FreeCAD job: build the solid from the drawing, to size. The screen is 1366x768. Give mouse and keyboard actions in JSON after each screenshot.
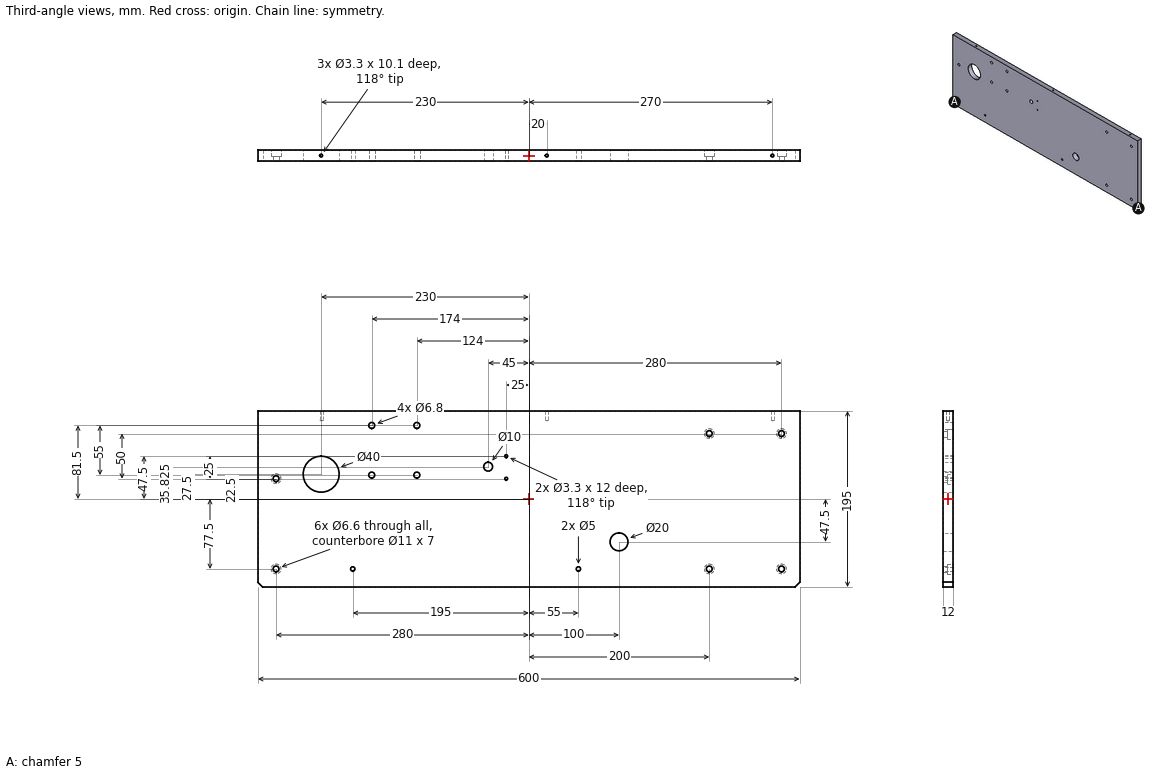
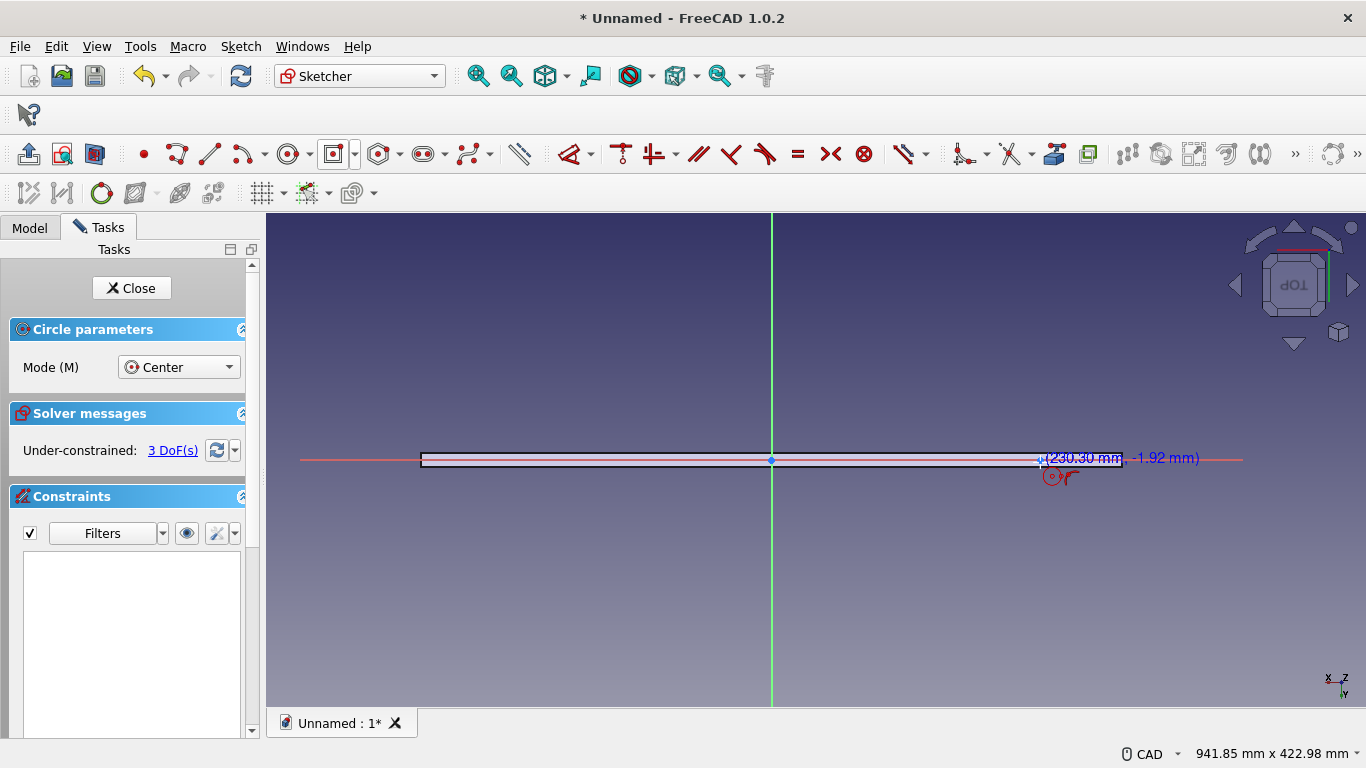
{"action": "scroll", "coordinate": [748, 460], "scroll_direction": "up", "scroll_amount": 13}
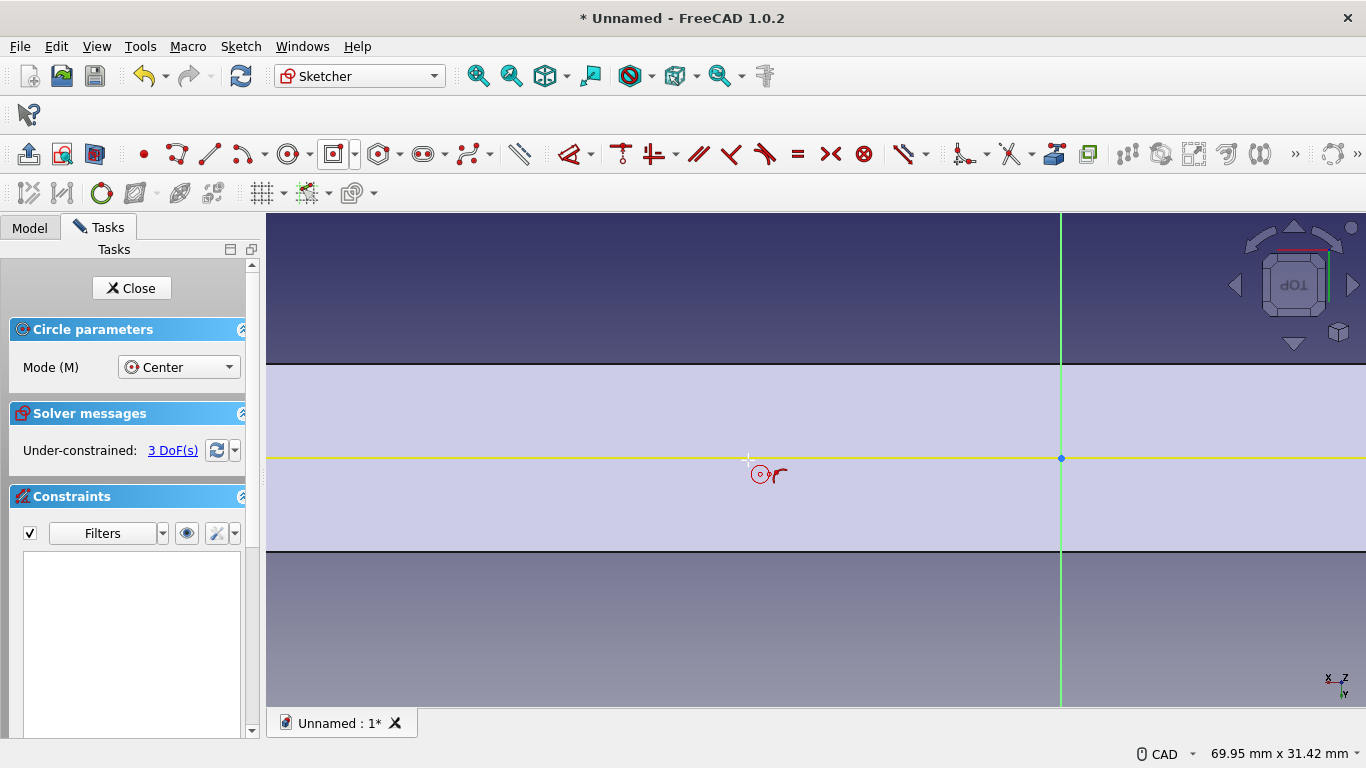
{"action": "scroll", "coordinate": [748, 460], "scroll_direction": "down", "scroll_amount": 13}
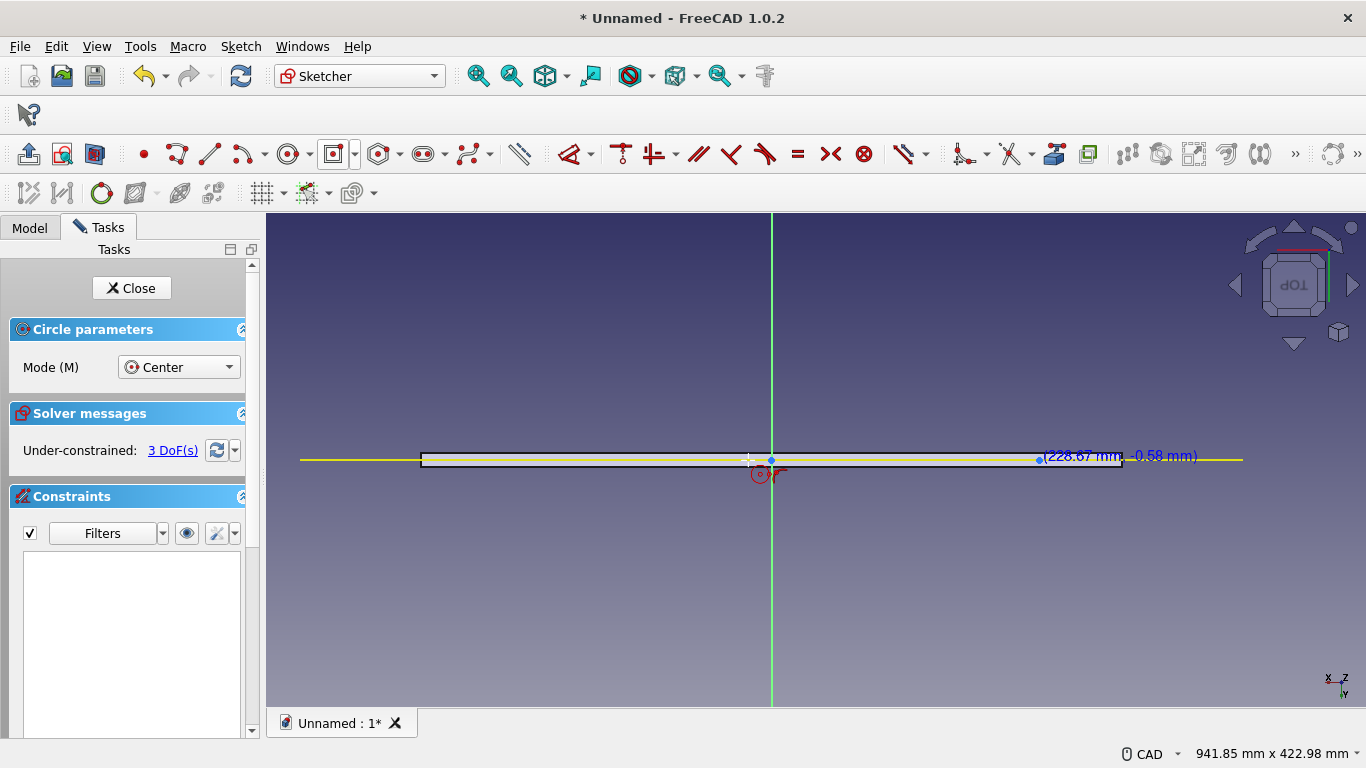
{"action": "left_click", "coordinate": [748, 460]}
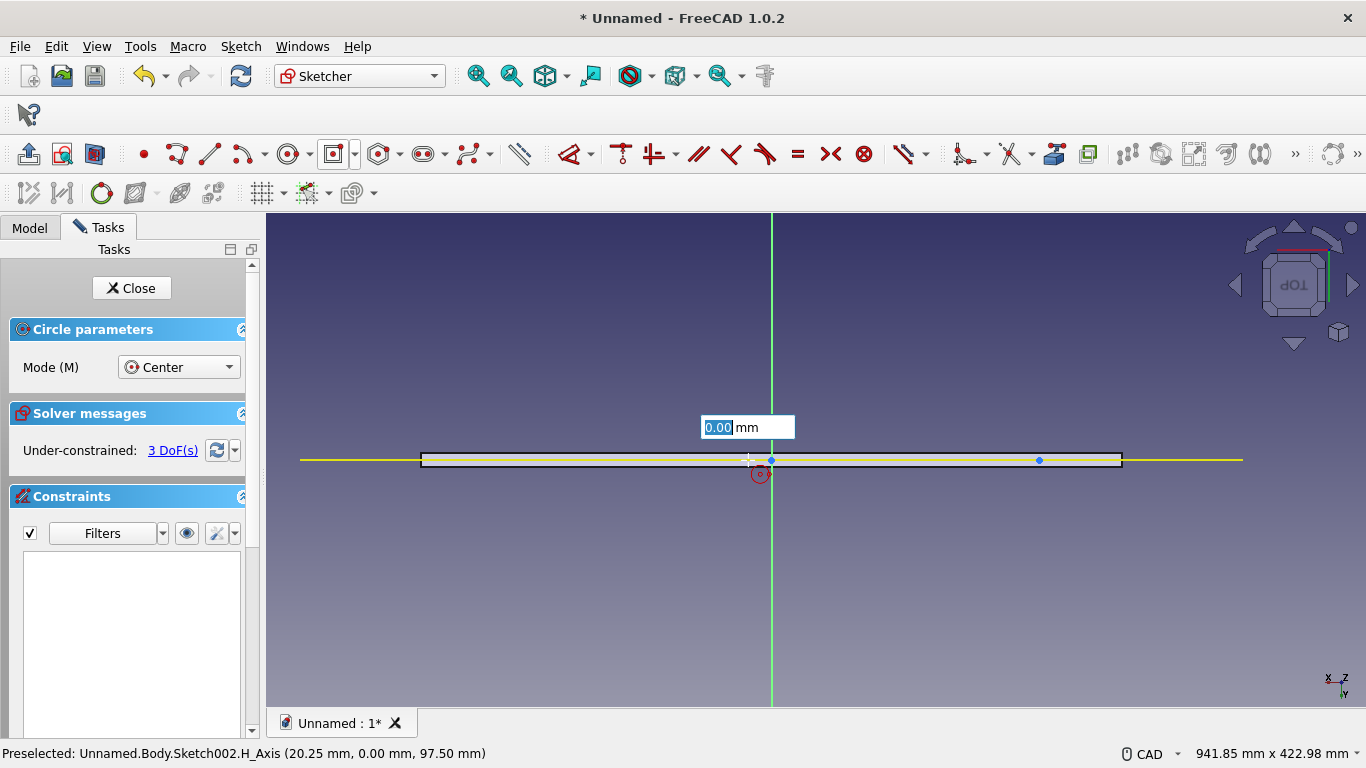
{"action": "scroll", "coordinate": [748, 462], "scroll_direction": "up", "scroll_amount": 11}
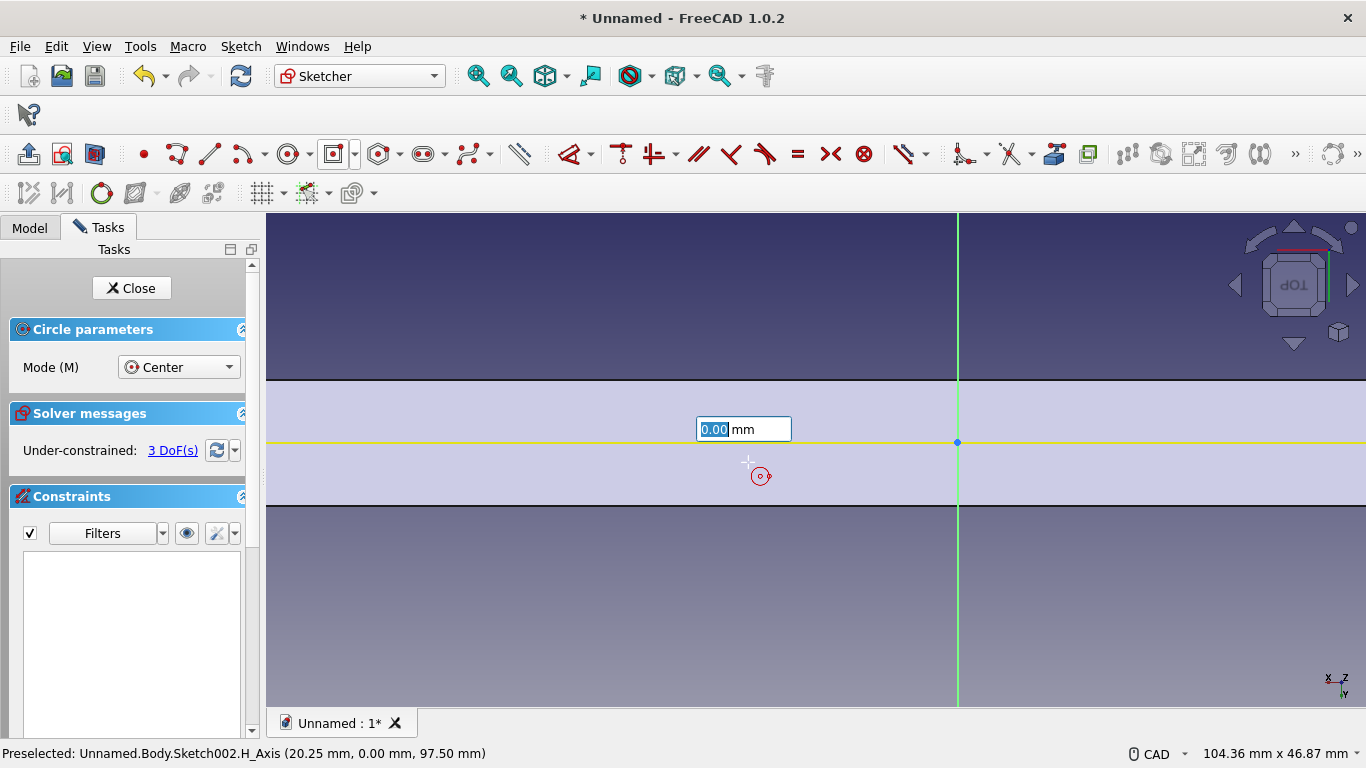
{"action": "left_click", "coordinate": [741, 459]}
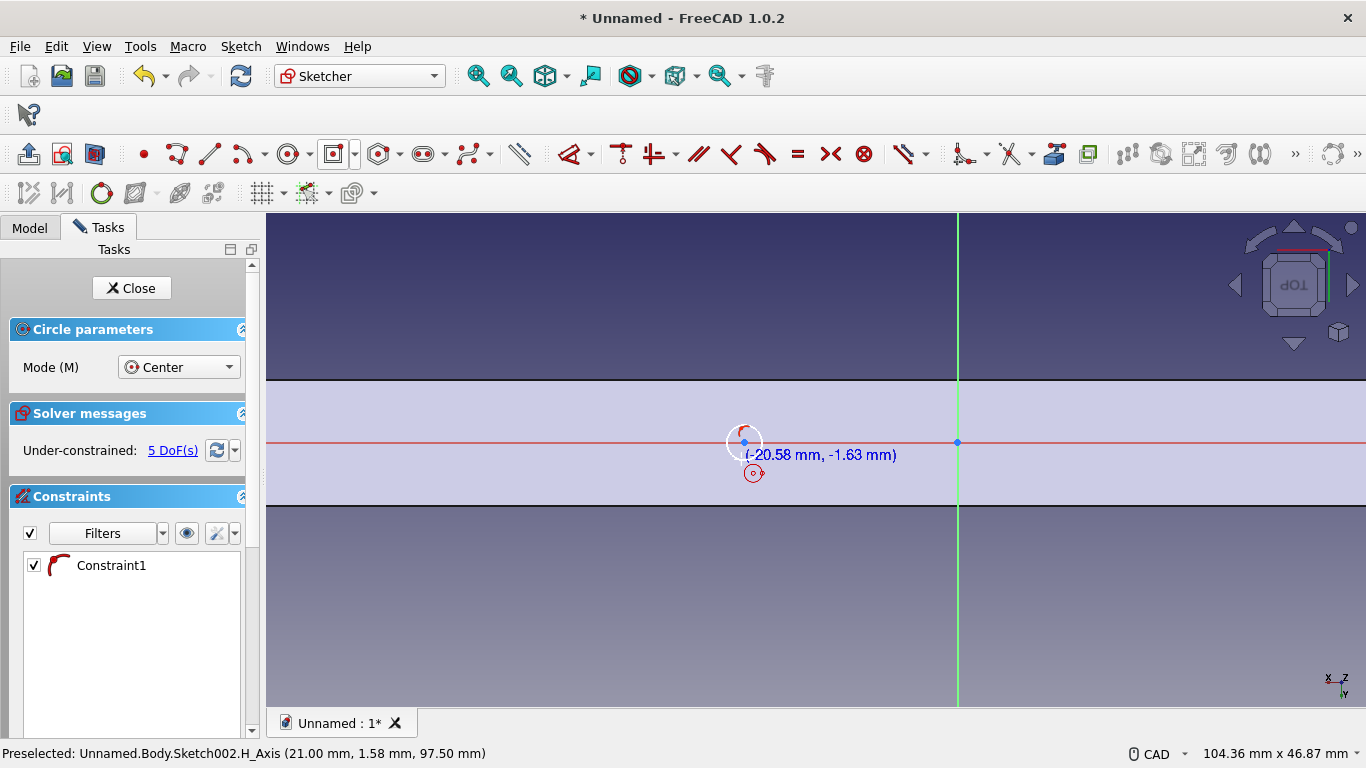
{"action": "scroll", "coordinate": [748, 462], "scroll_direction": "down", "scroll_amount": 11}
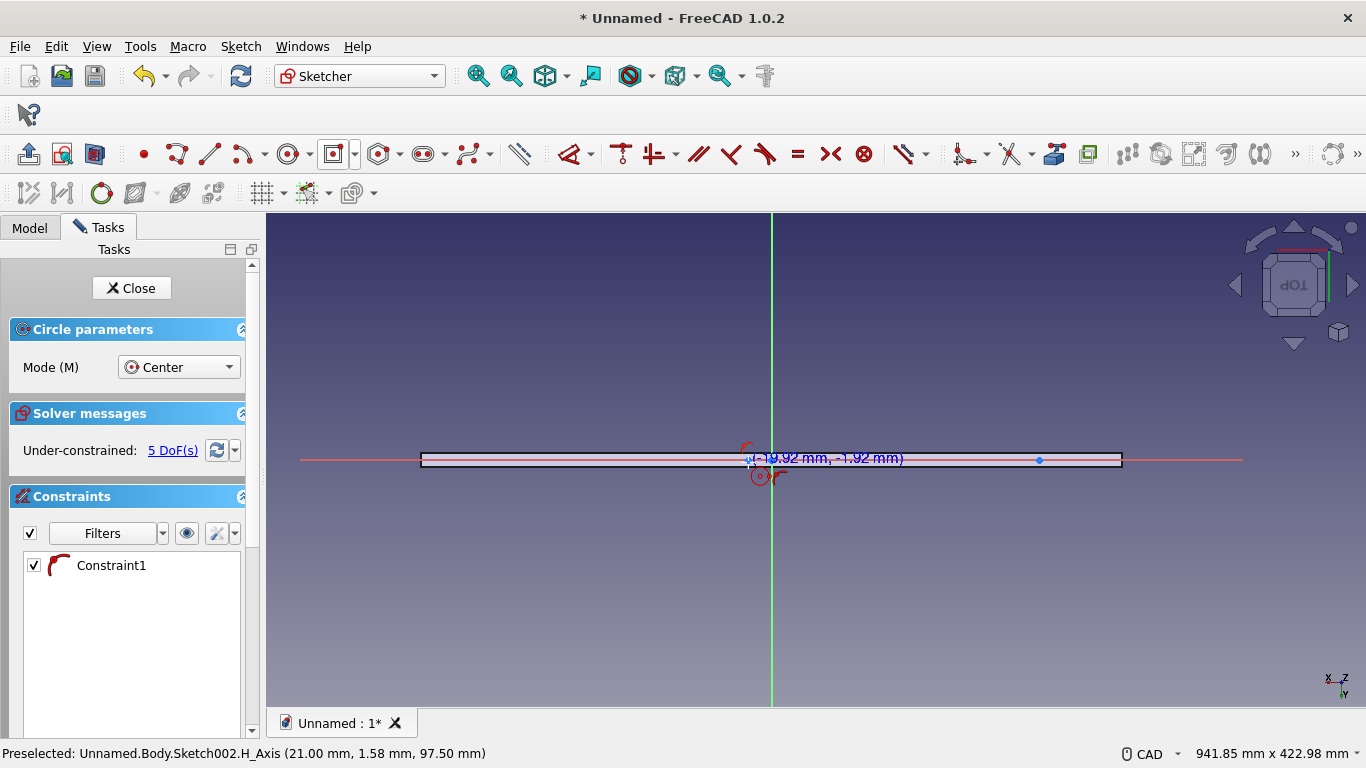
{"action": "scroll", "coordinate": [456, 460], "scroll_direction": "up", "scroll_amount": 13}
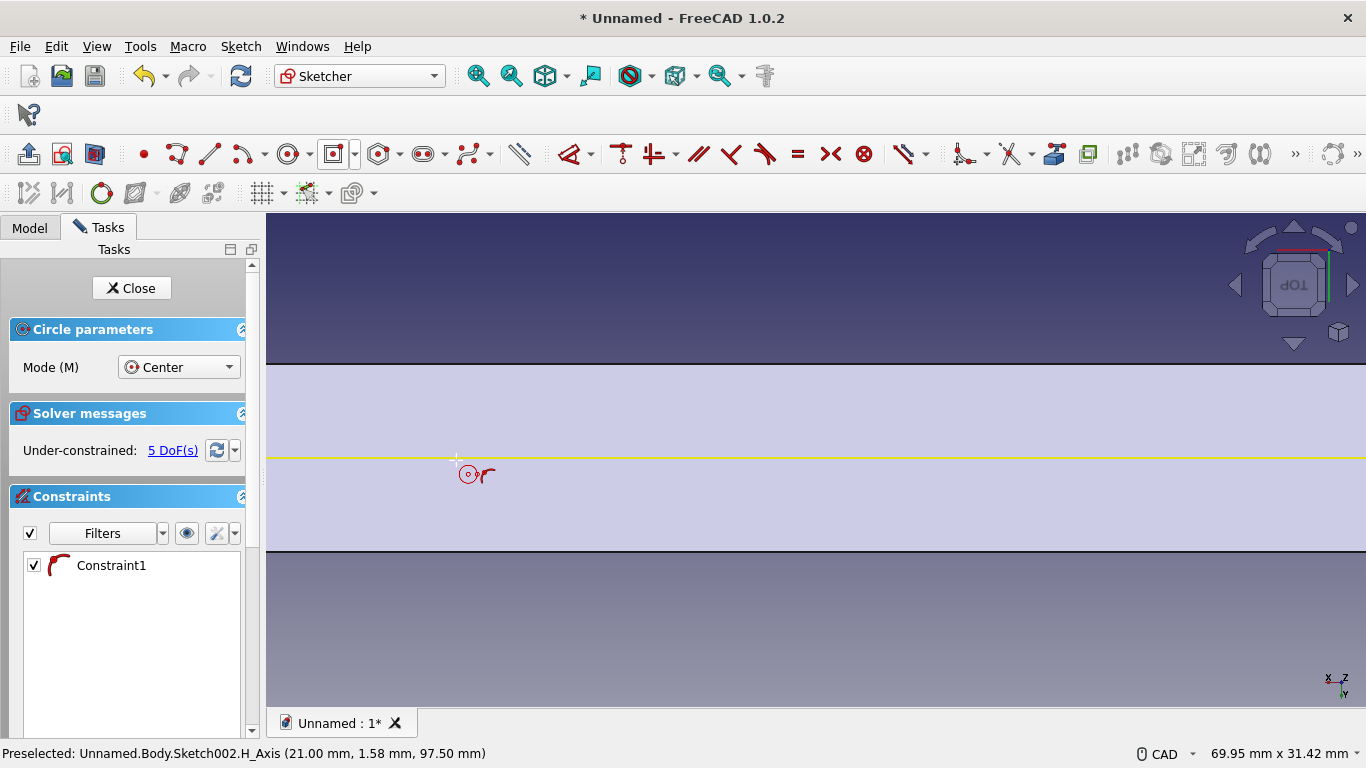
{"action": "scroll", "coordinate": [455, 460], "scroll_direction": "down", "scroll_amount": 13}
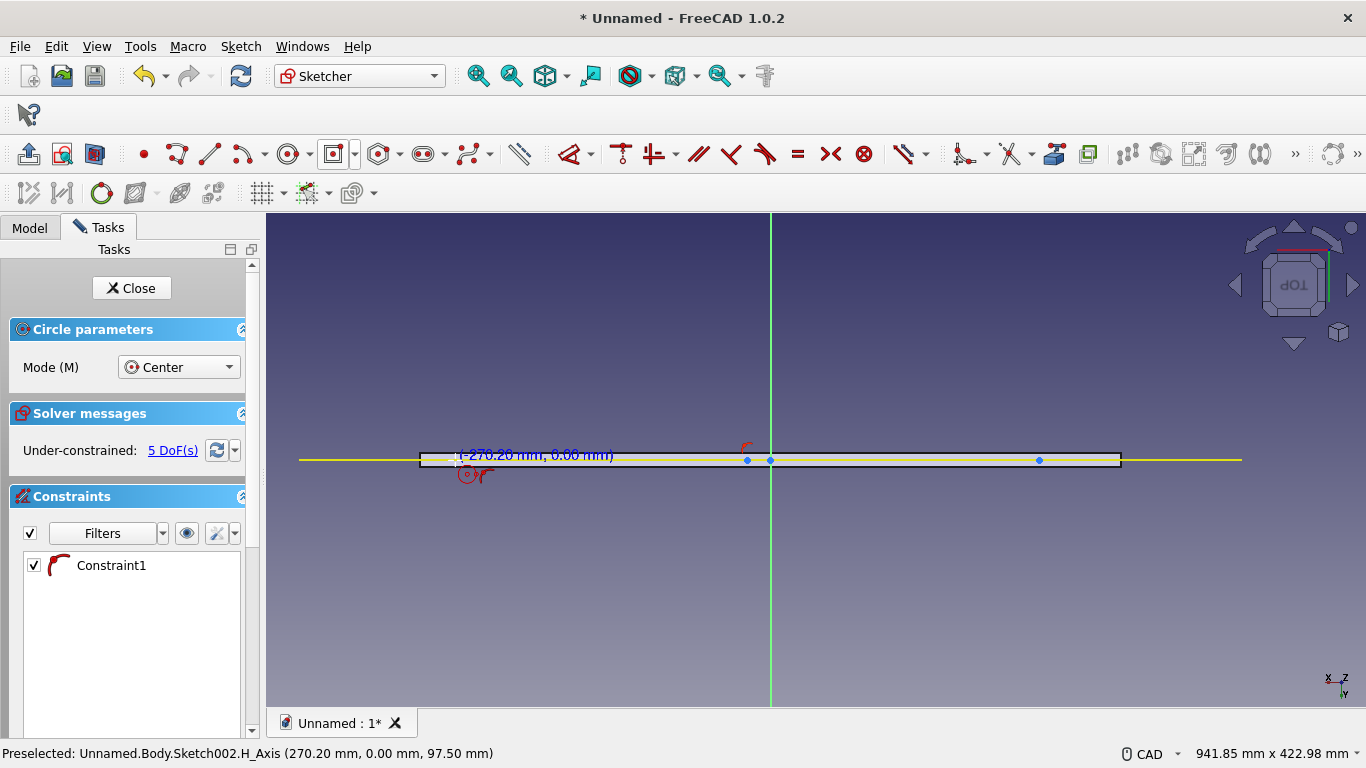
{"action": "left_click", "coordinate": [455, 460]}